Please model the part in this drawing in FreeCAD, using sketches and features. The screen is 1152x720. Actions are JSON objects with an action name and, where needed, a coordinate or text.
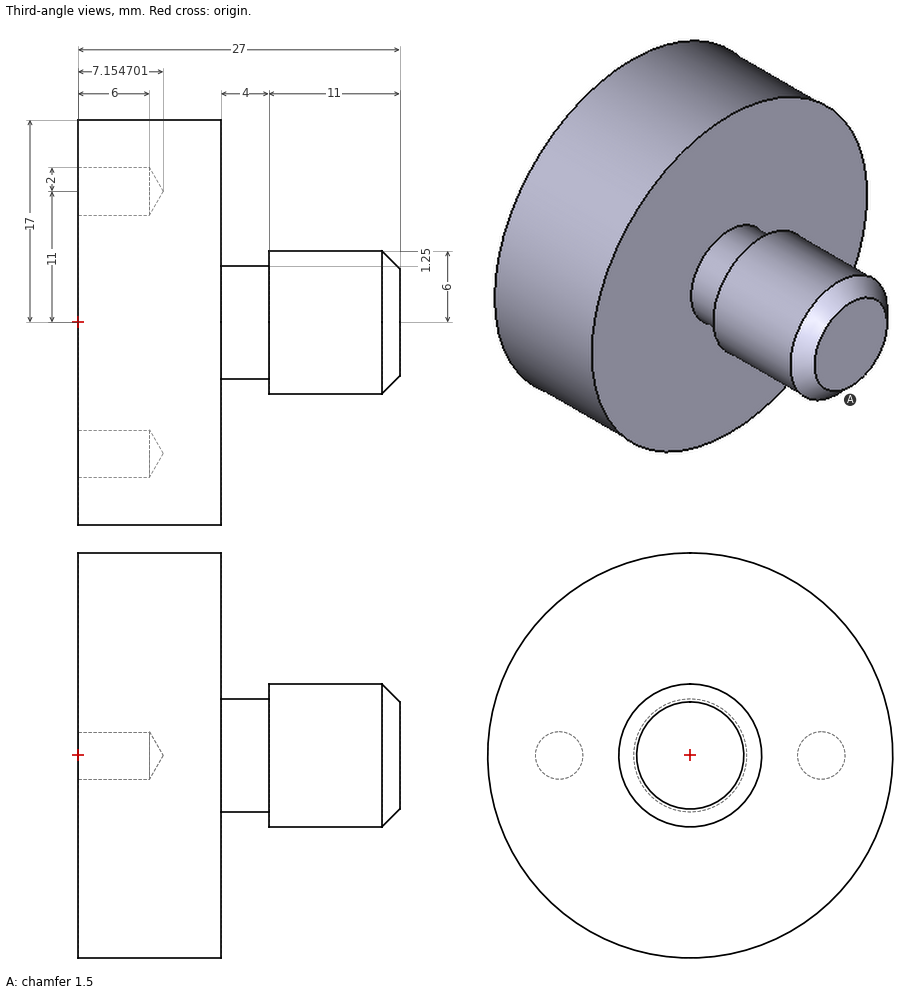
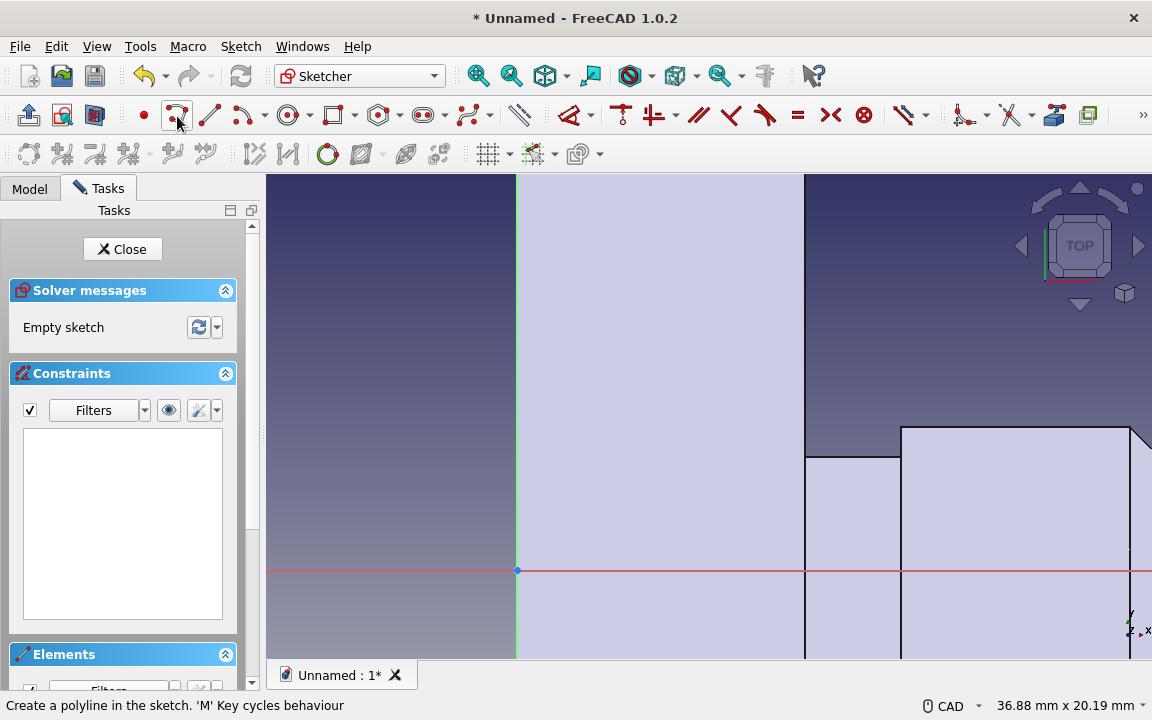
{"action": "left_click", "coordinate": [517, 307]}
{"action": "left_click", "coordinate": [689, 307]}
{"action": "left_click", "coordinate": [661, 259]}
{"action": "left_click", "coordinate": [526, 259]}
{"action": "left_click", "coordinate": [517, 308]}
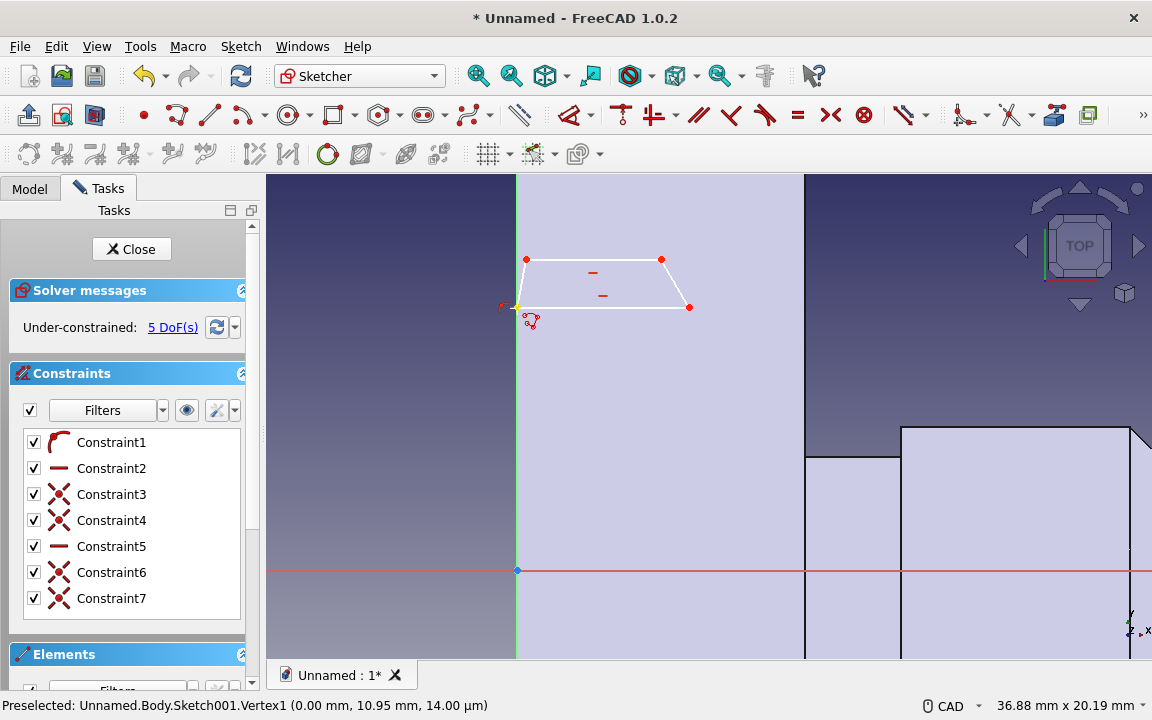
{"action": "left_click", "coordinate": [210, 116]}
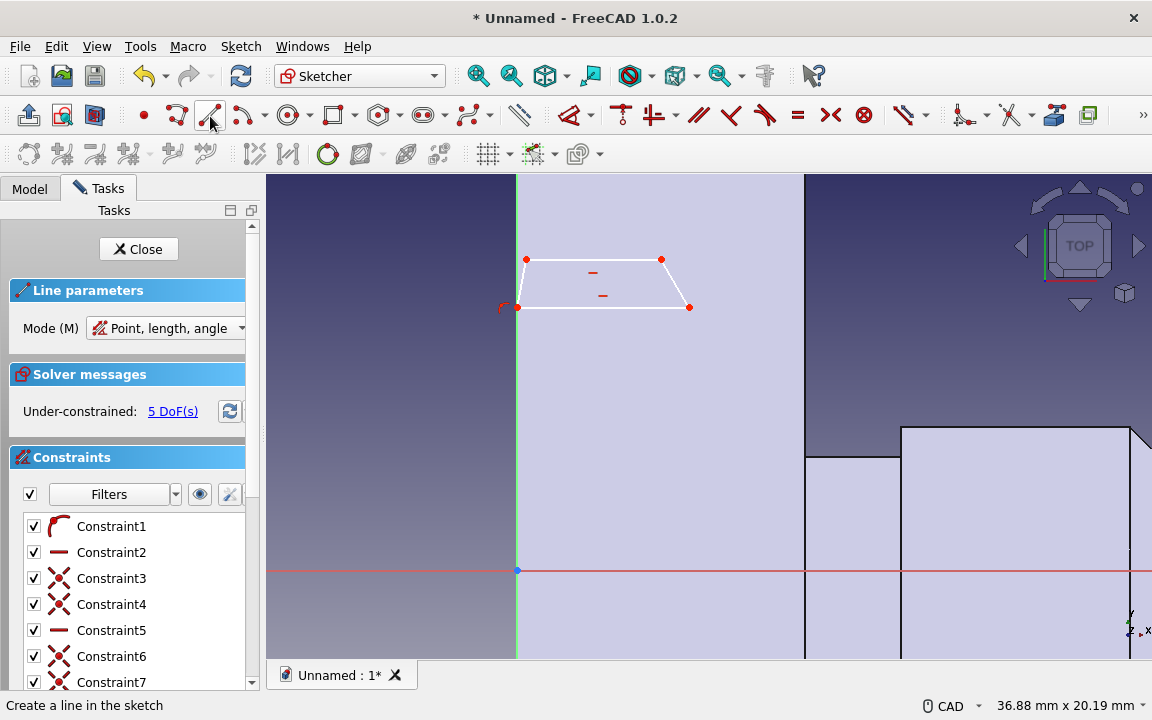
{"action": "left_click", "coordinate": [706, 307]}
{"action": "left_click", "coordinate": [758, 307]}
{"action": "key", "text": "Escape"}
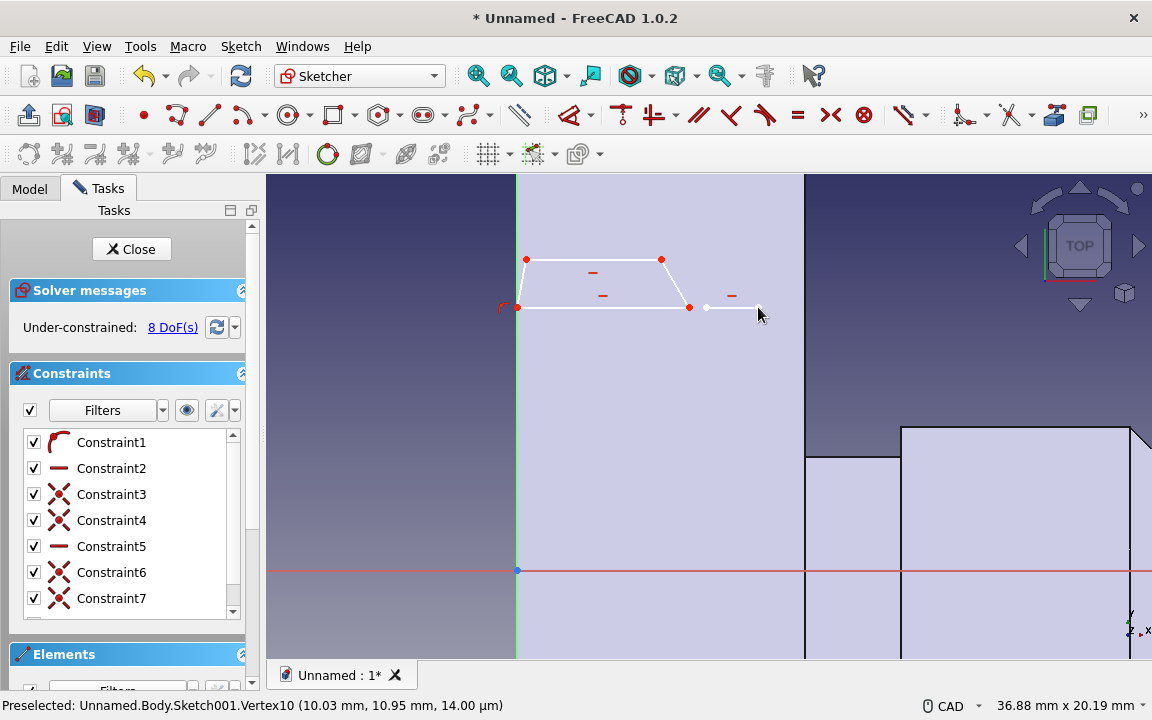
{"action": "left_click", "coordinate": [722, 308]}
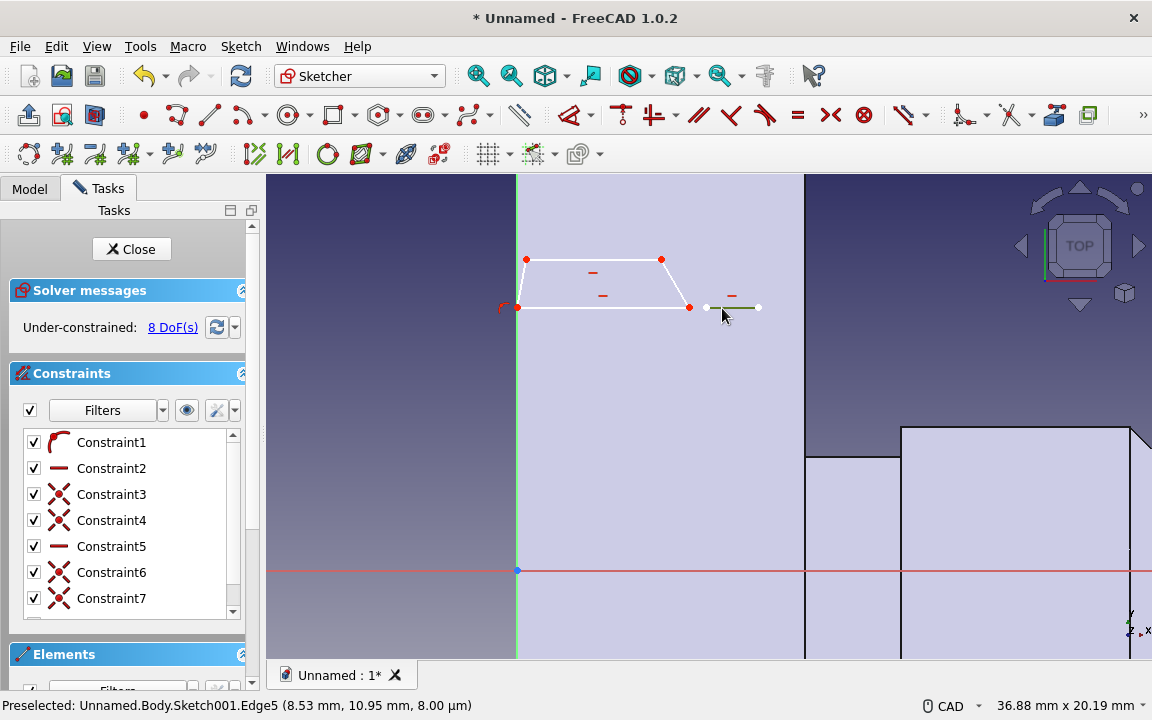
{"action": "left_click", "coordinate": [520, 116]}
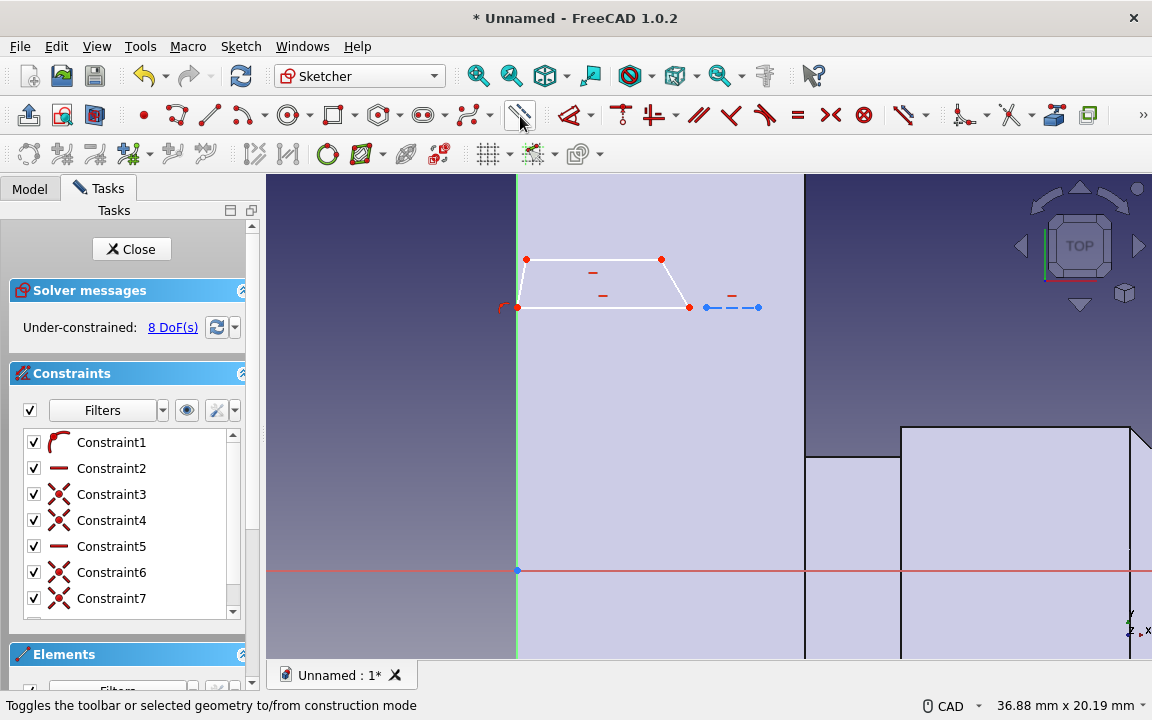
{"action": "left_click", "coordinate": [520, 294]}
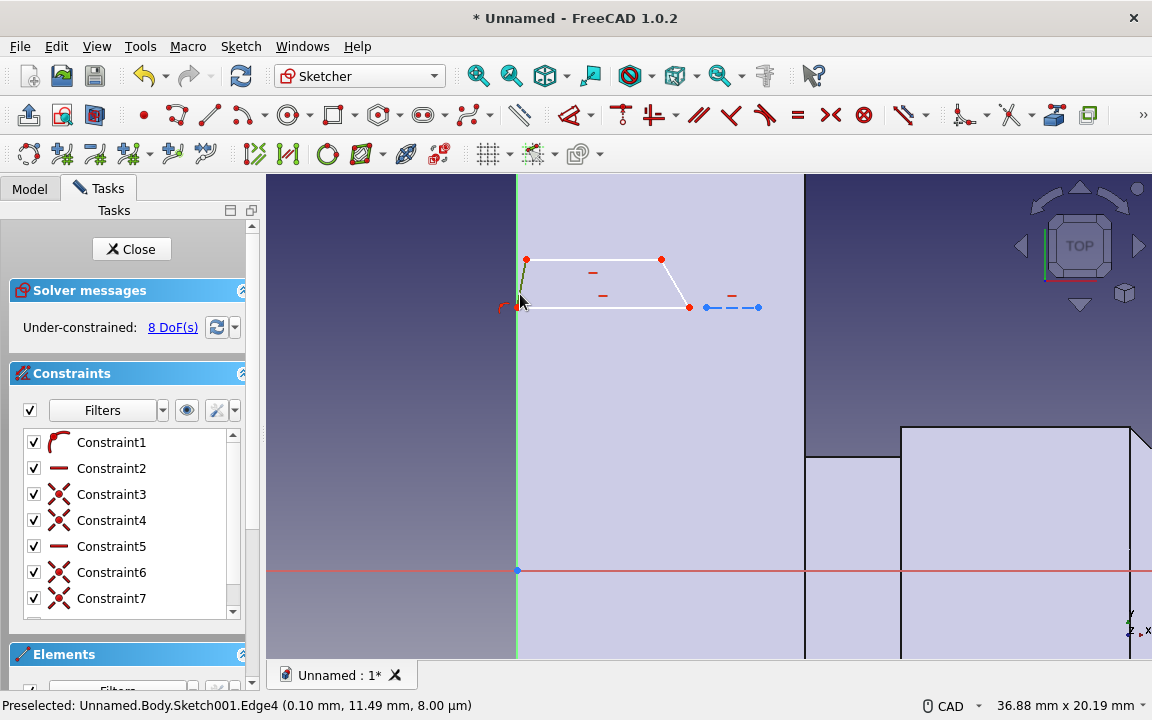
{"action": "key", "text": "v"}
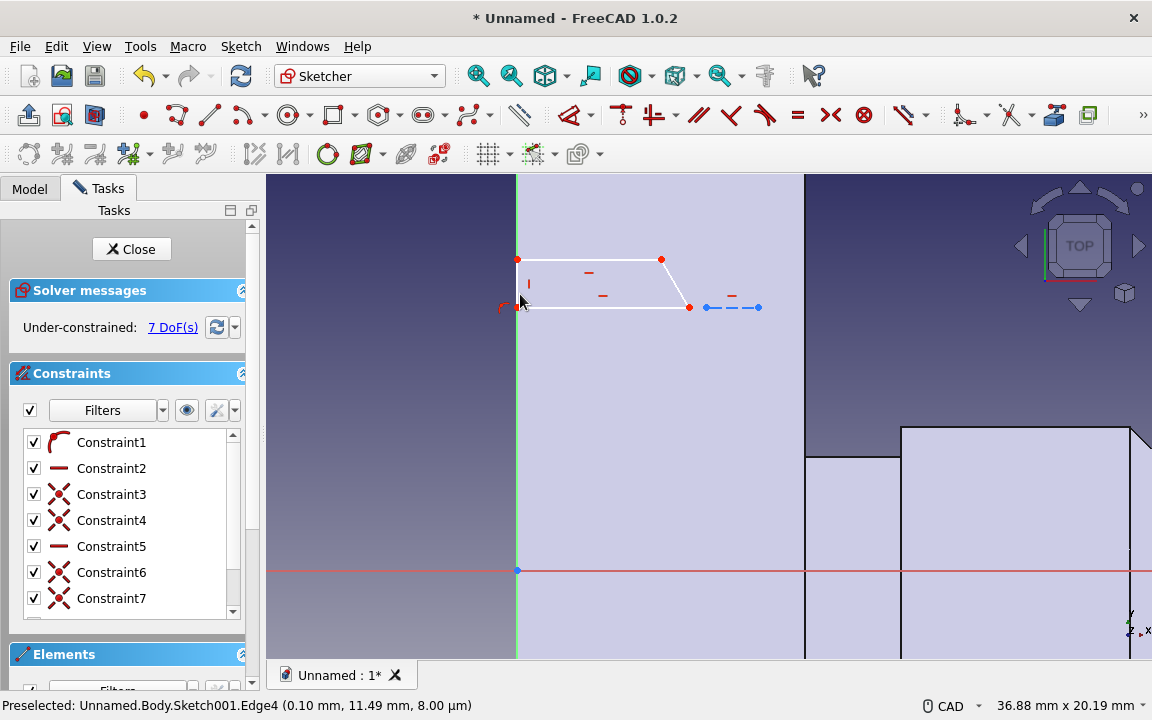
{"action": "left_click", "coordinate": [568, 116]}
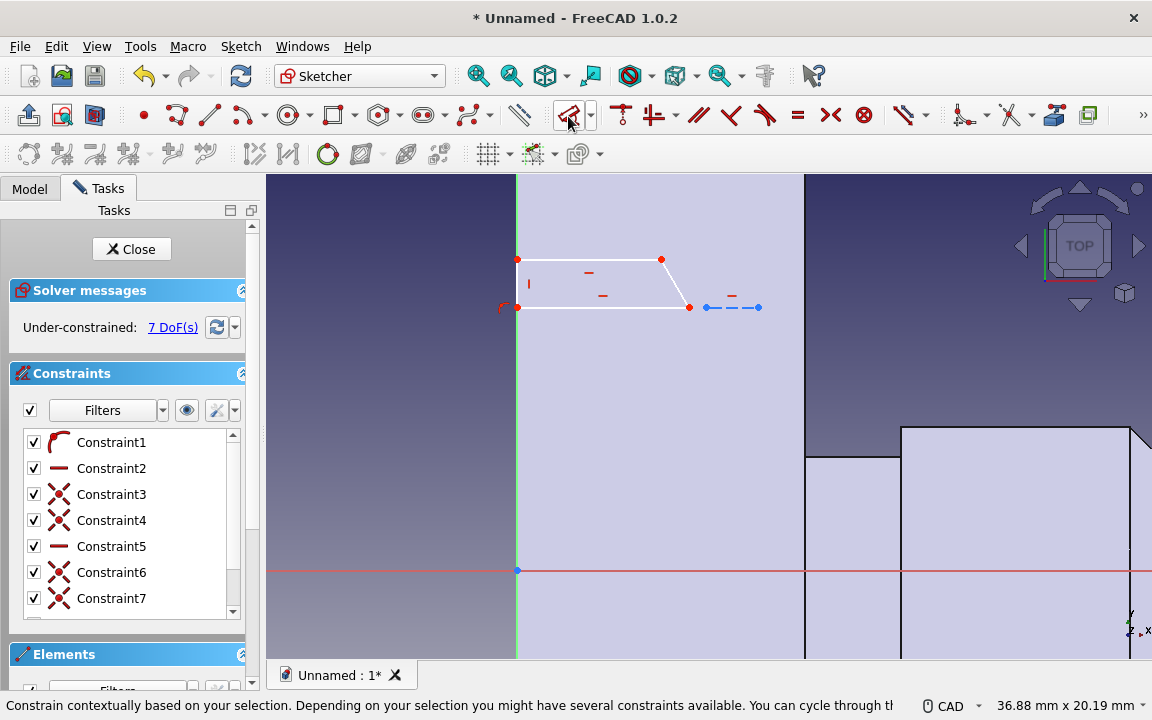
{"action": "left_click", "coordinate": [618, 260]}
{"action": "left_click", "coordinate": [589, 226]}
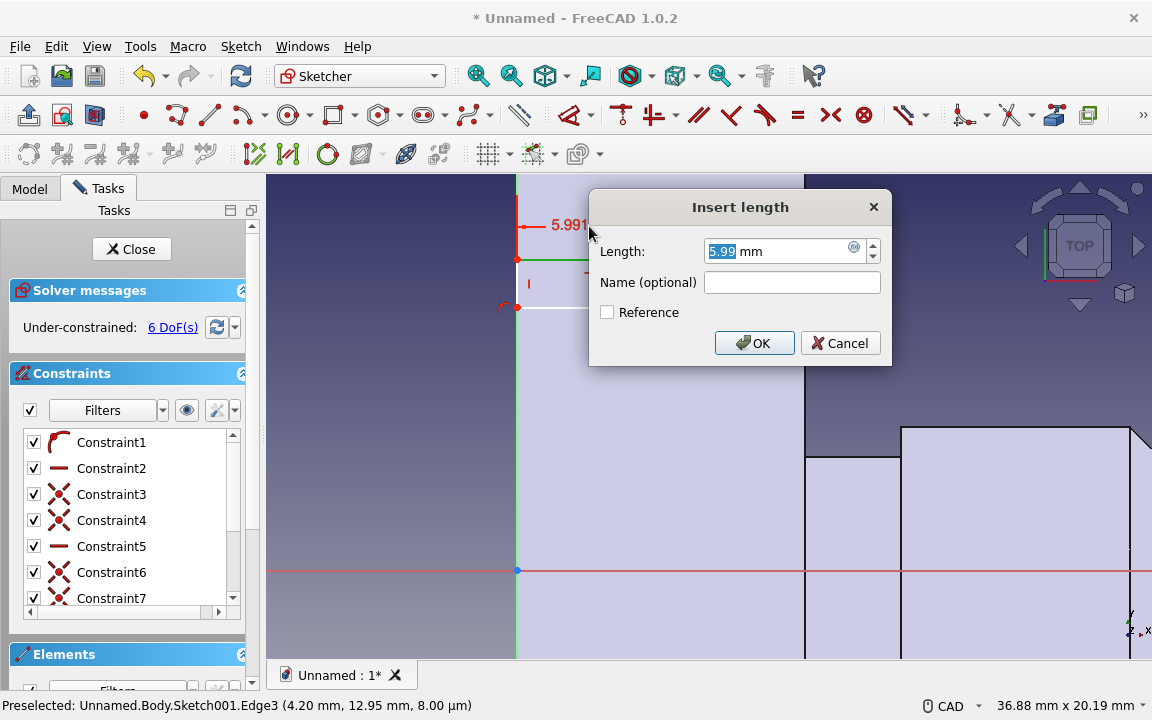
{"action": "type", "text": "6"}
{"action": "key", "text": "Return"}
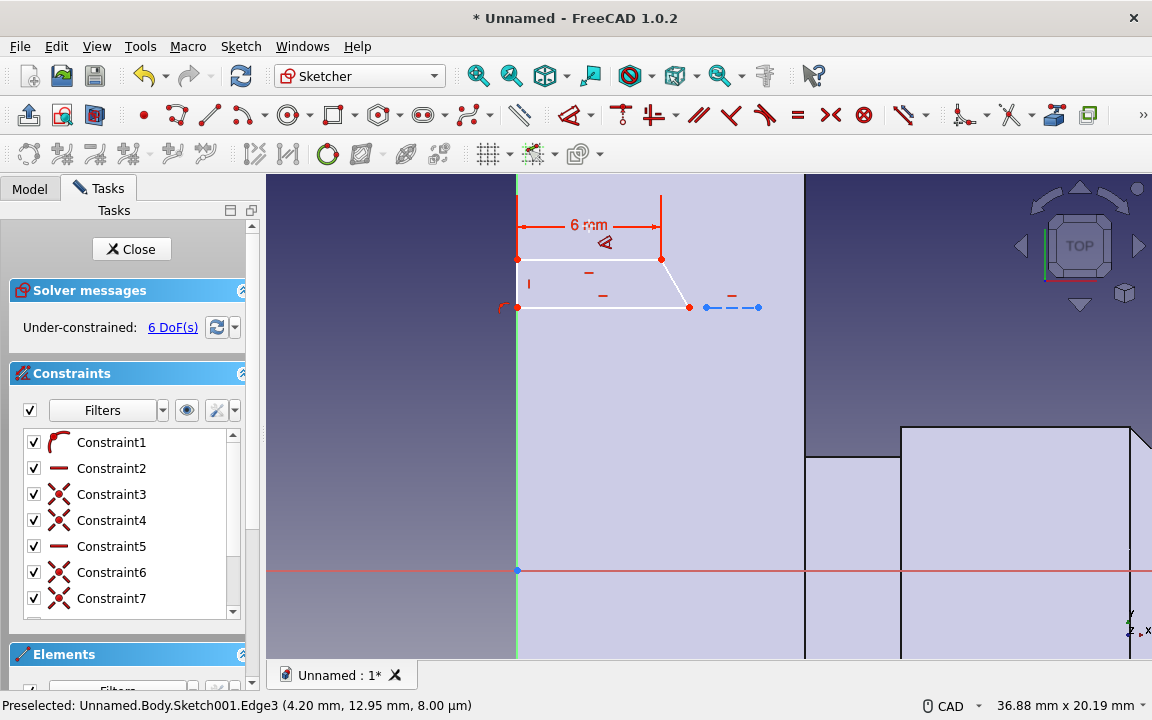
{"action": "left_click", "coordinate": [517, 274]}
{"action": "left_click", "coordinate": [483, 284]}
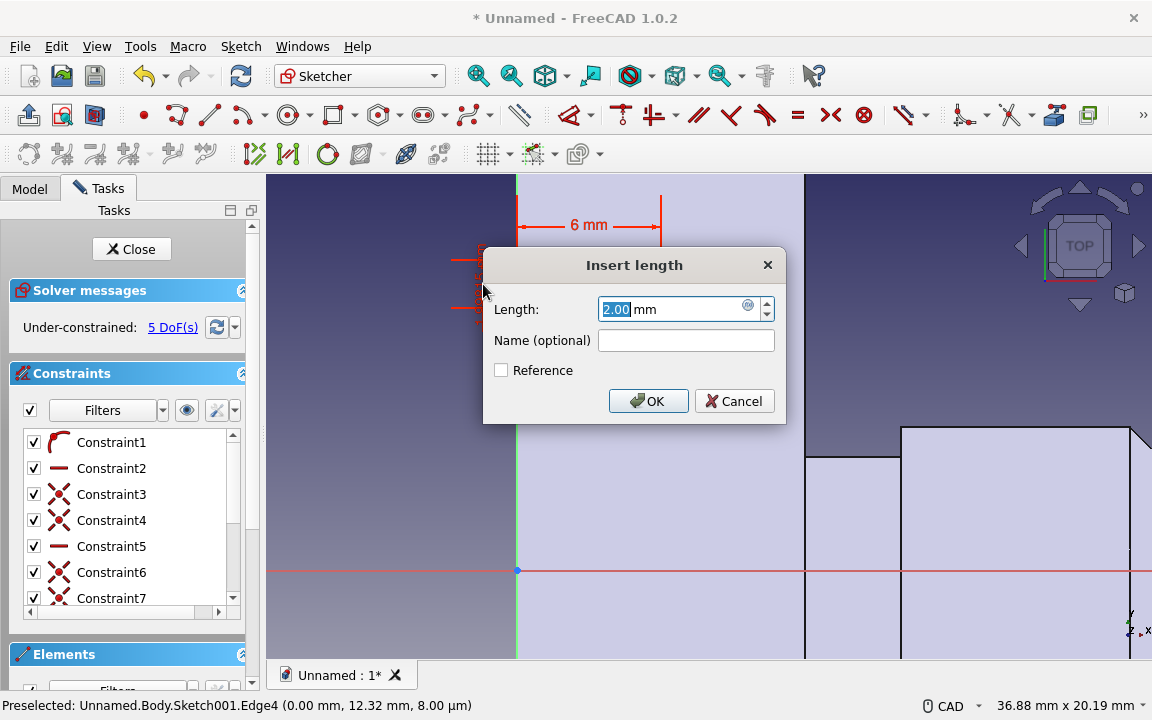
{"action": "type", "text": "2"}
{"action": "key", "text": "Return"}